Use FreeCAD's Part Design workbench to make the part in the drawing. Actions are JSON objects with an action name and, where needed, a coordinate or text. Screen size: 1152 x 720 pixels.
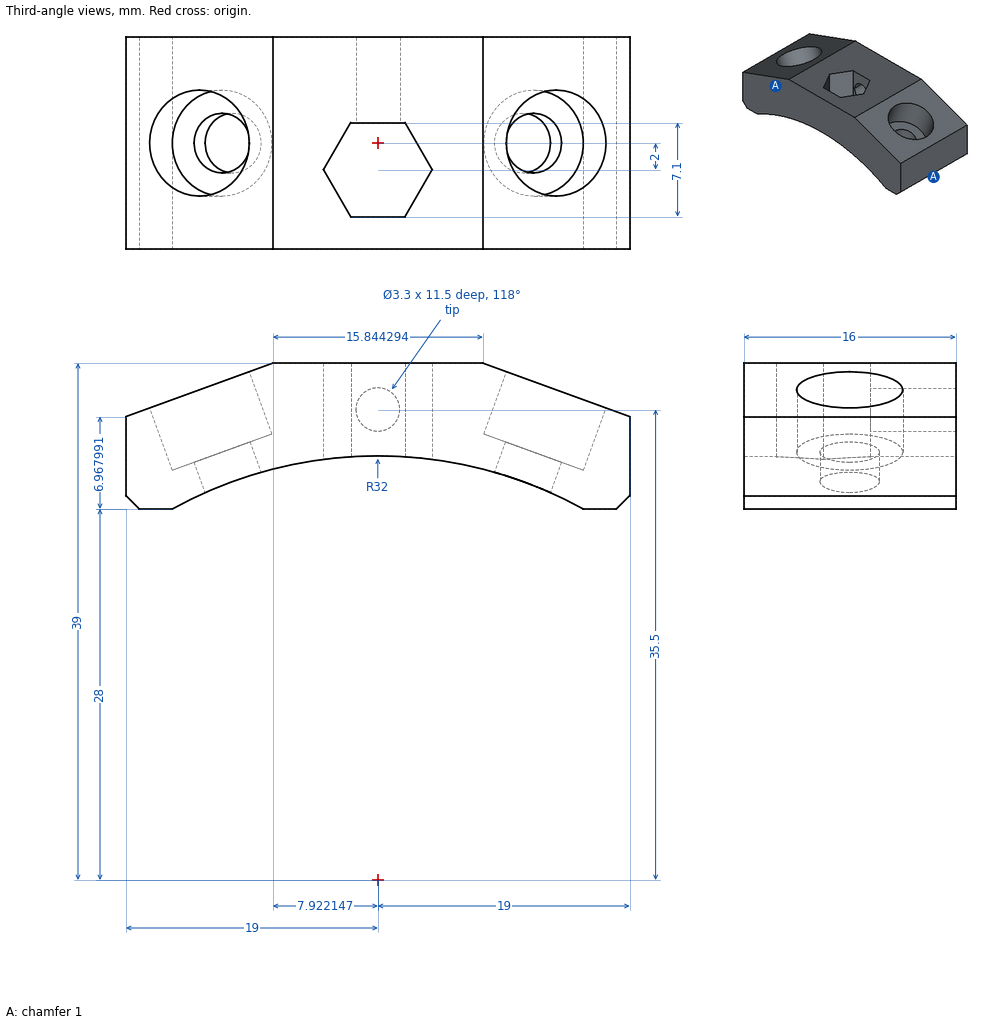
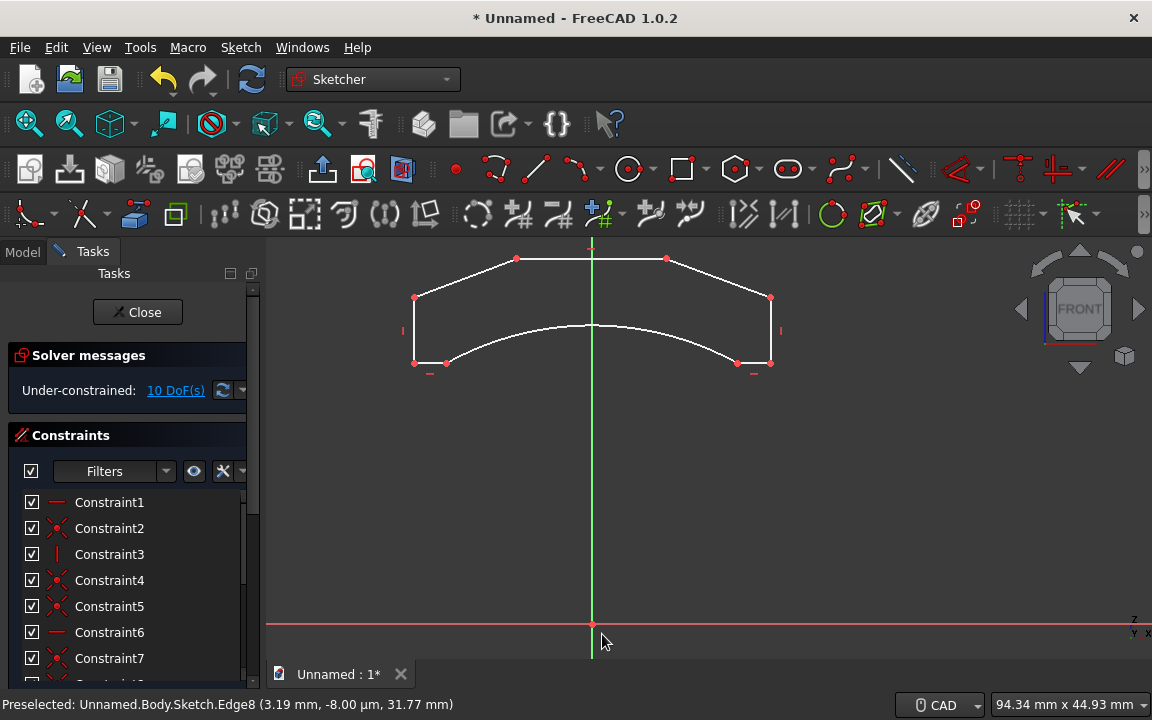
{"action": "key", "text": "d"}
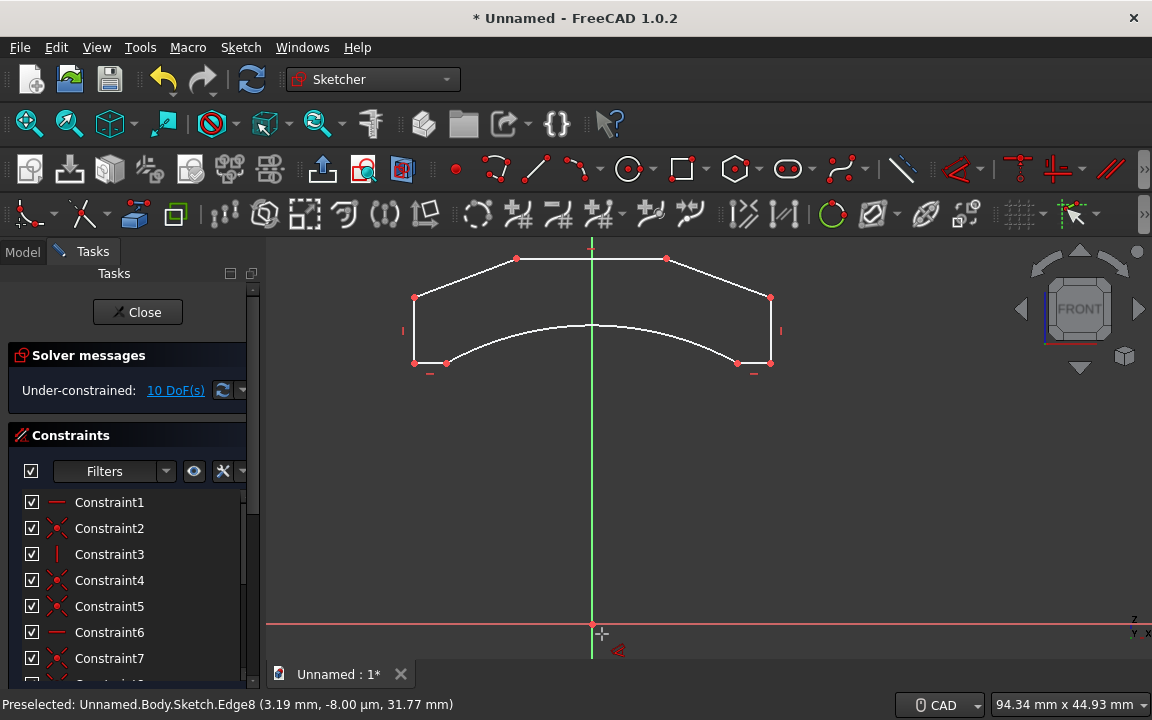
{"action": "left_click", "coordinate": [653, 332]}
{"action": "left_click", "coordinate": [660, 301]}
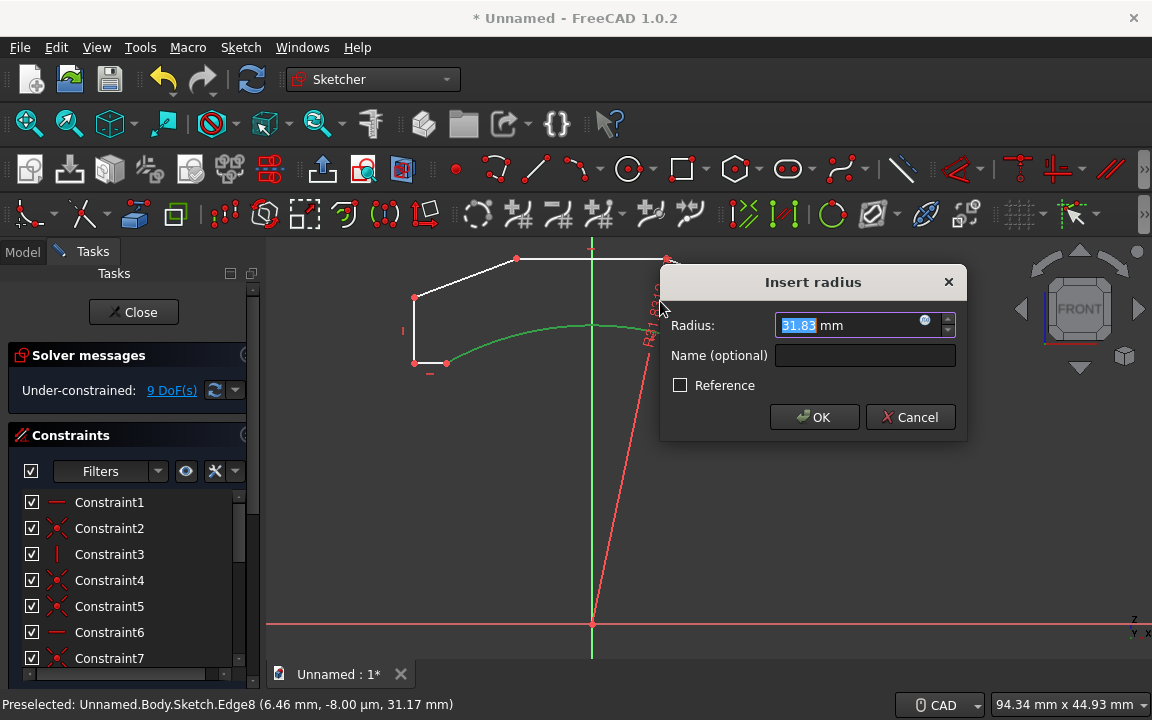
{"action": "type", "text": "32"}
{"action": "key", "text": "Return"}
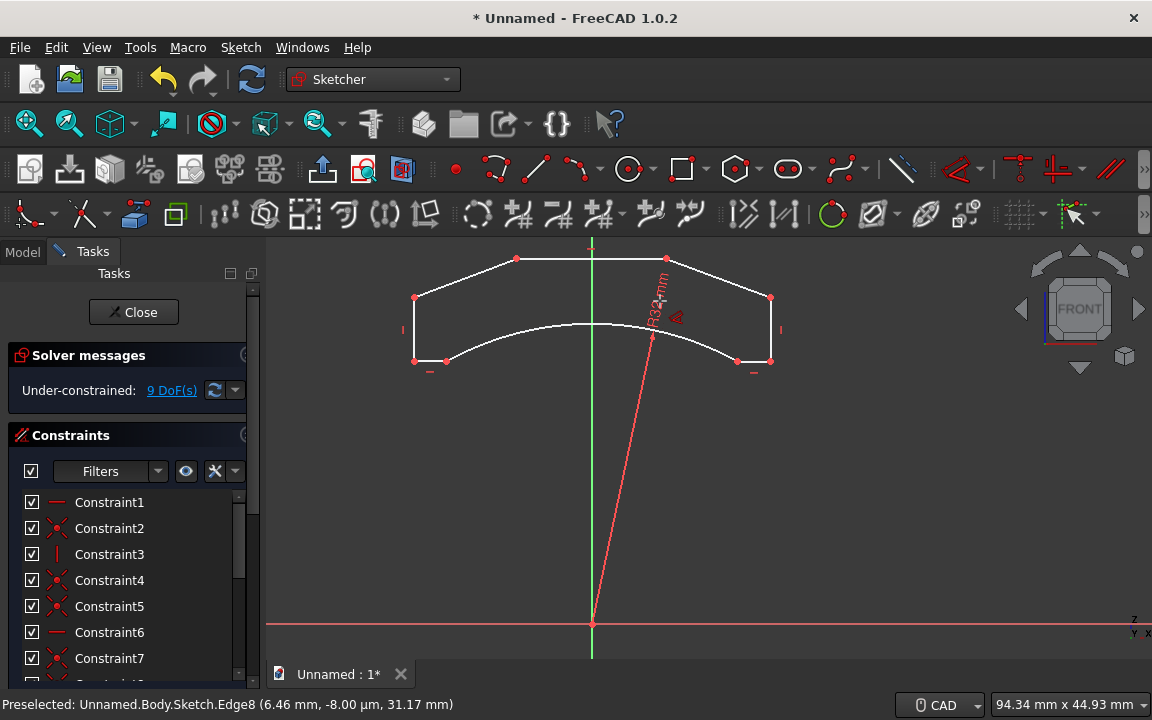
{"action": "left_click", "coordinate": [447, 361]}
{"action": "left_click", "coordinate": [413, 493]}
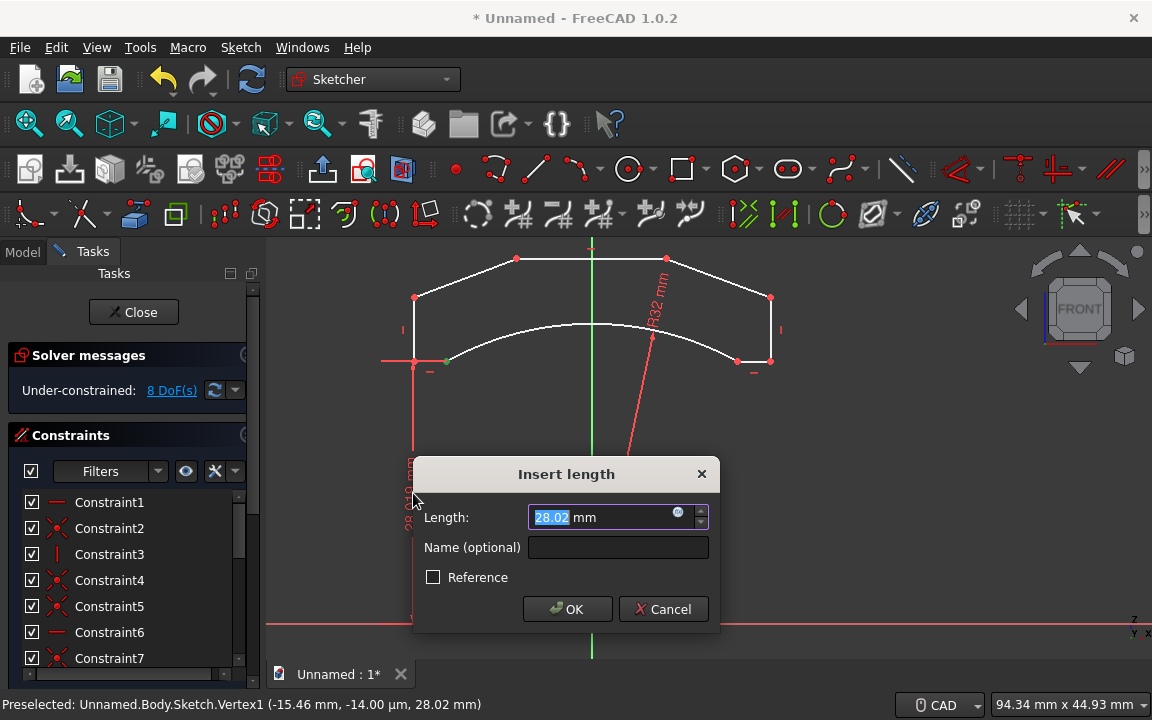
{"action": "type", "text": "28"}
{"action": "key", "text": "Return"}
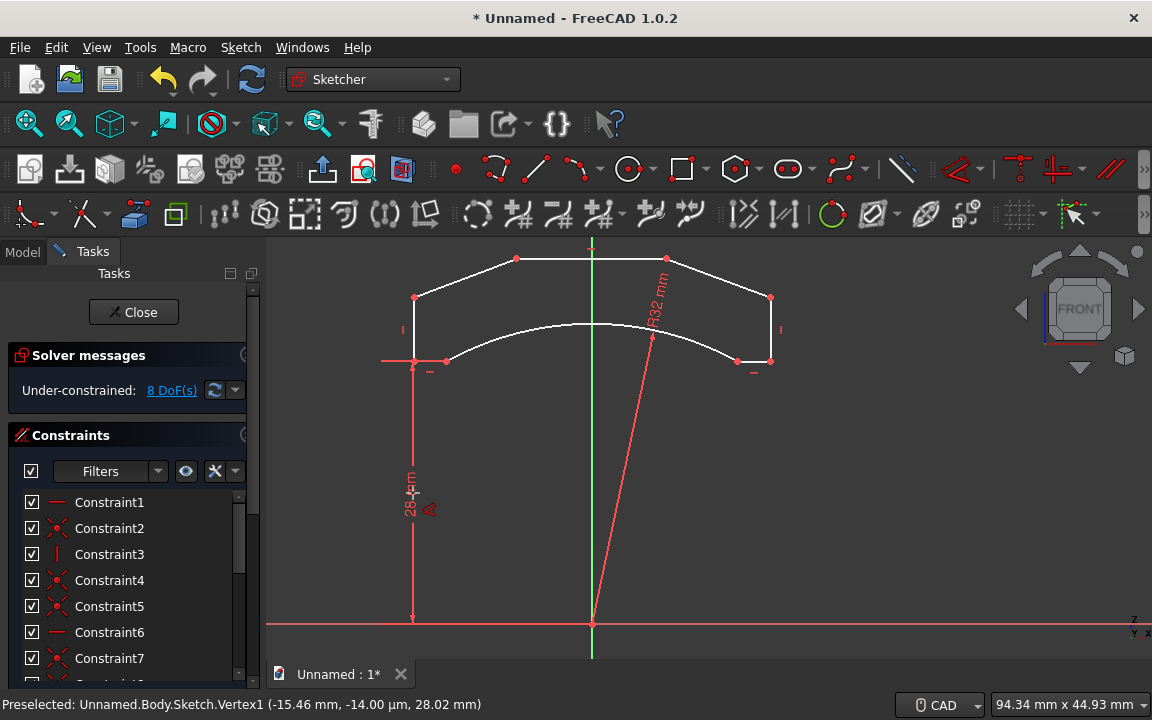
{"action": "left_click", "coordinate": [414, 361]}
{"action": "left_click", "coordinate": [462, 327]}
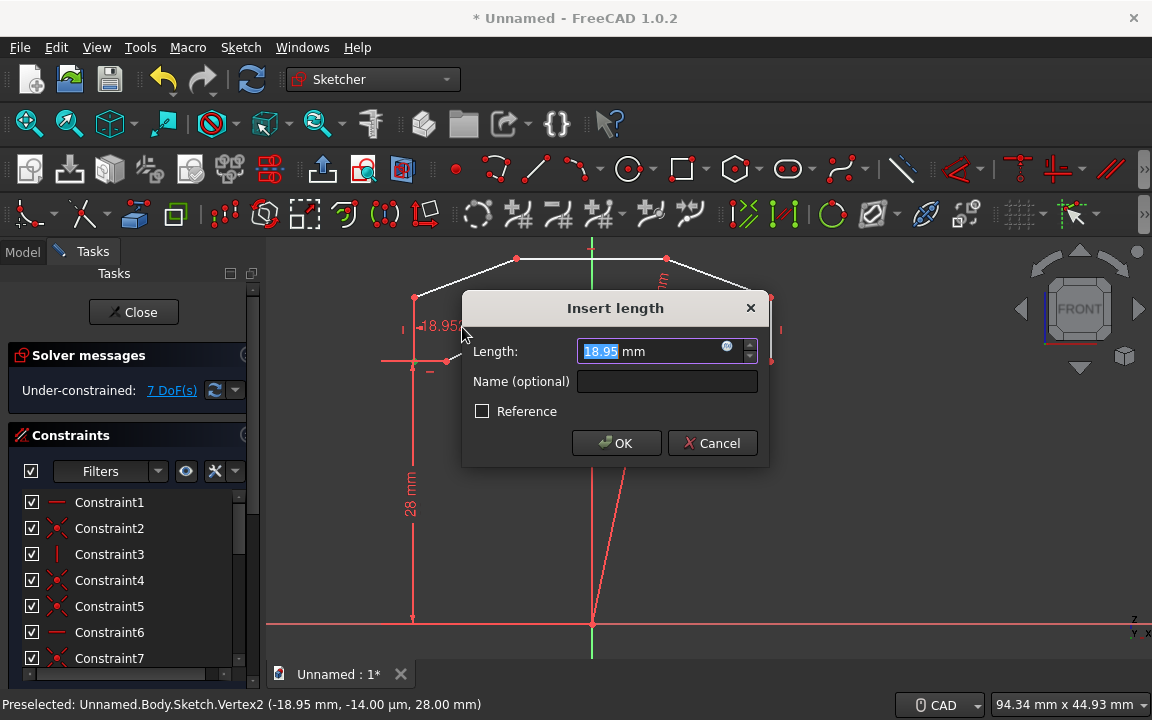
{"action": "type", "text": "19"}
{"action": "key", "text": "Return"}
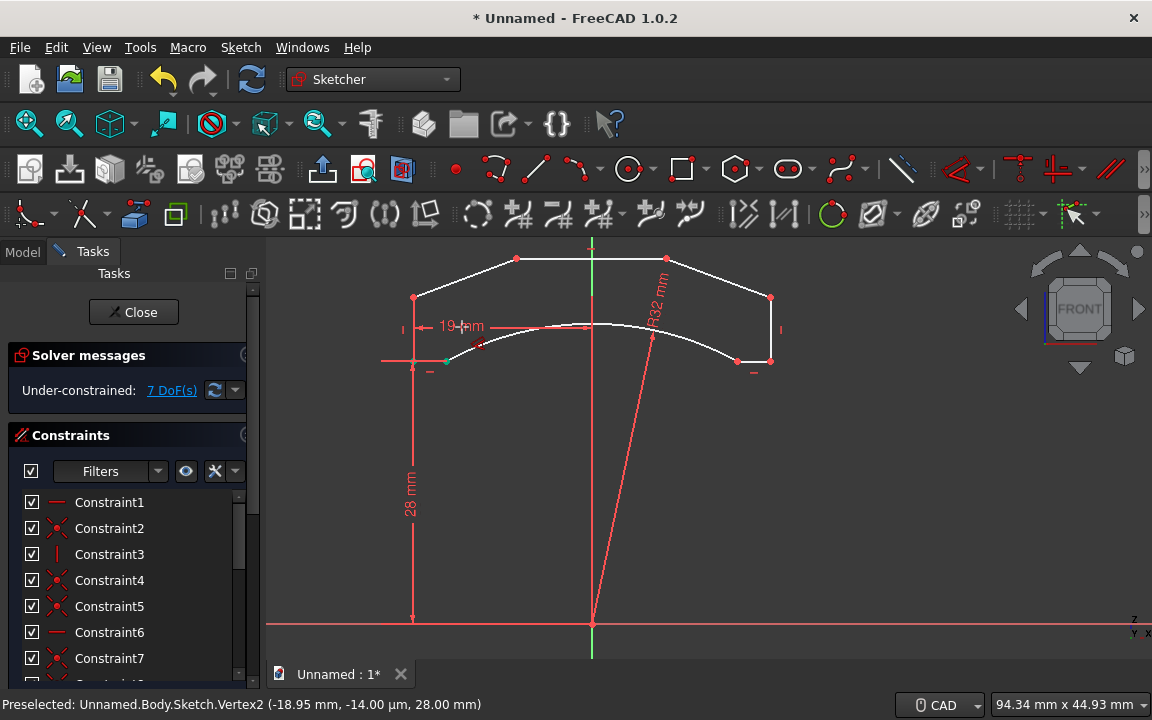
{"action": "scroll", "coordinate": [739, 462], "scroll_direction": "down", "scroll_amount": 2}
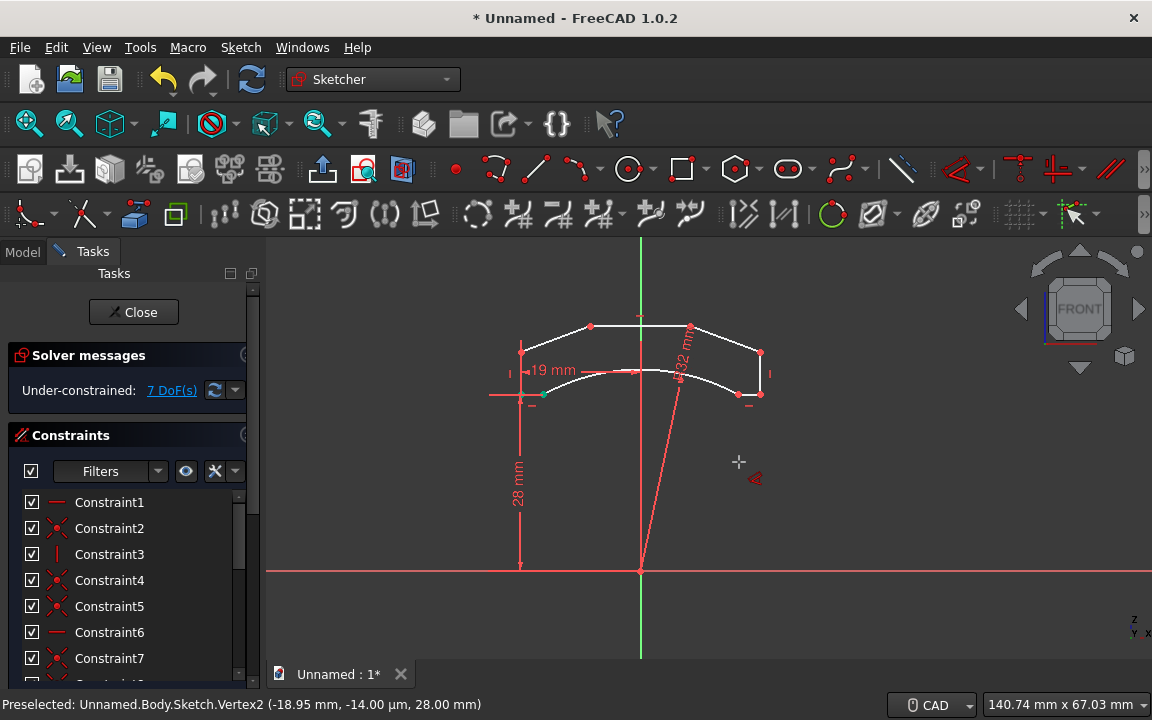
{"action": "left_click", "coordinate": [590, 326]}
{"action": "left_click", "coordinate": [556, 449]}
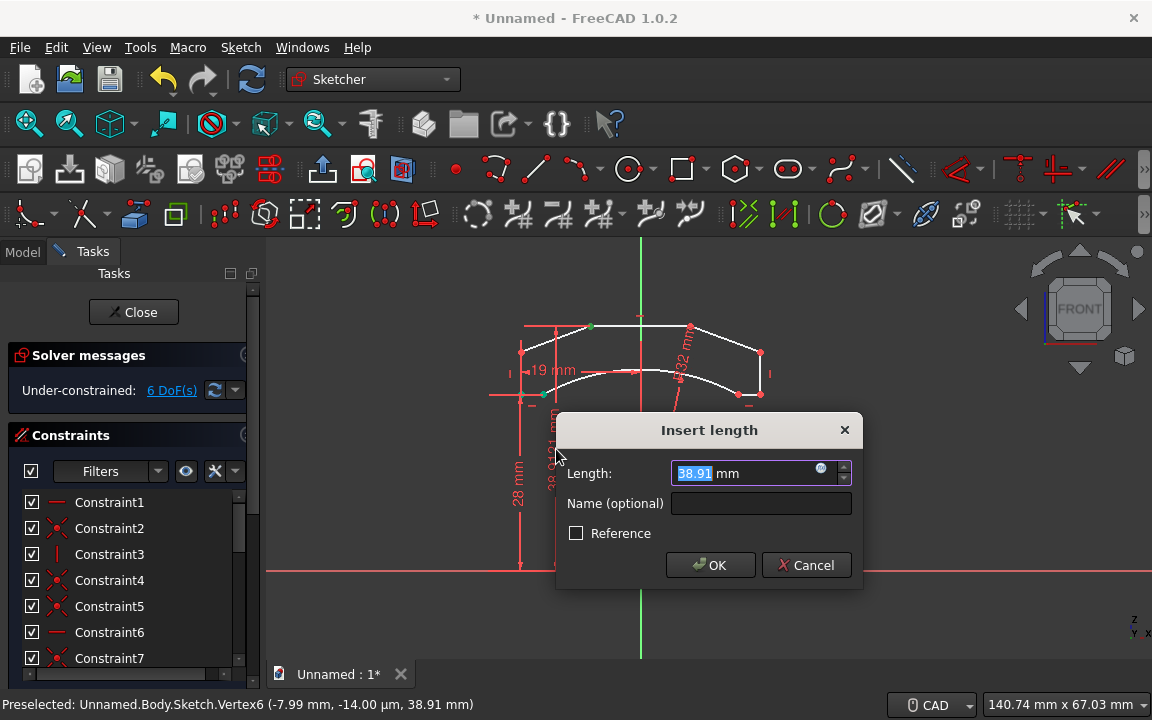
{"action": "type", "text": "39"}
{"action": "key", "text": "Return"}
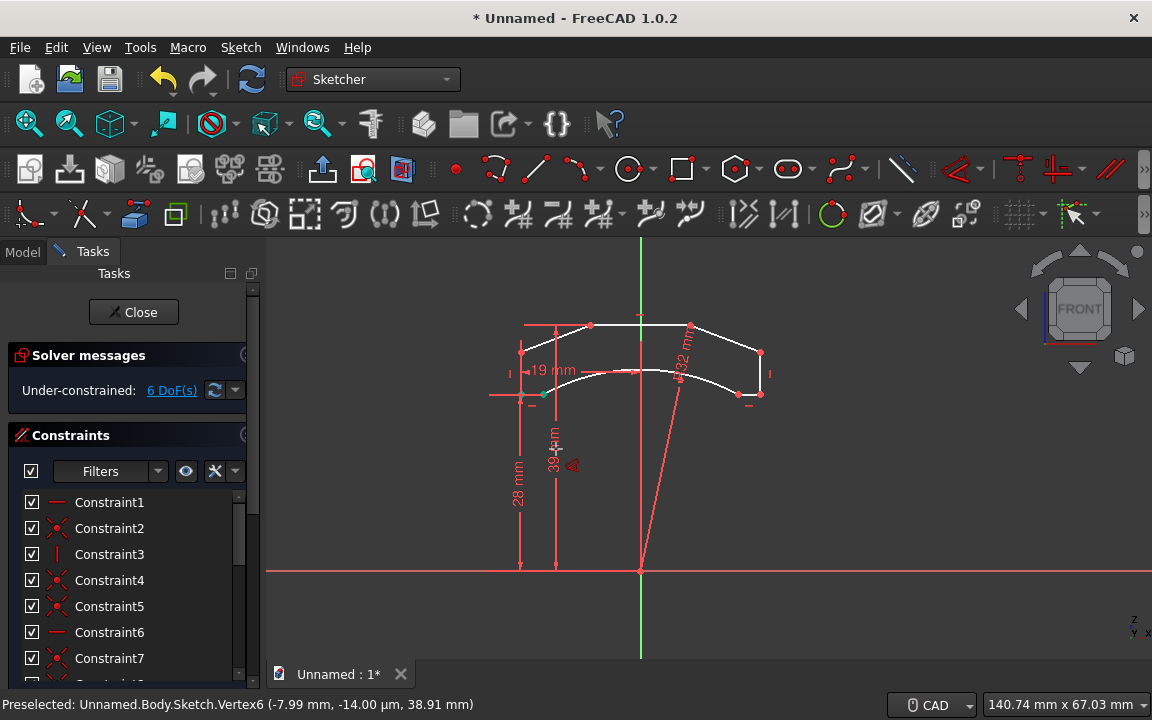
{"action": "left_click", "coordinate": [760, 352]}
{"action": "left_click", "coordinate": [700, 605]}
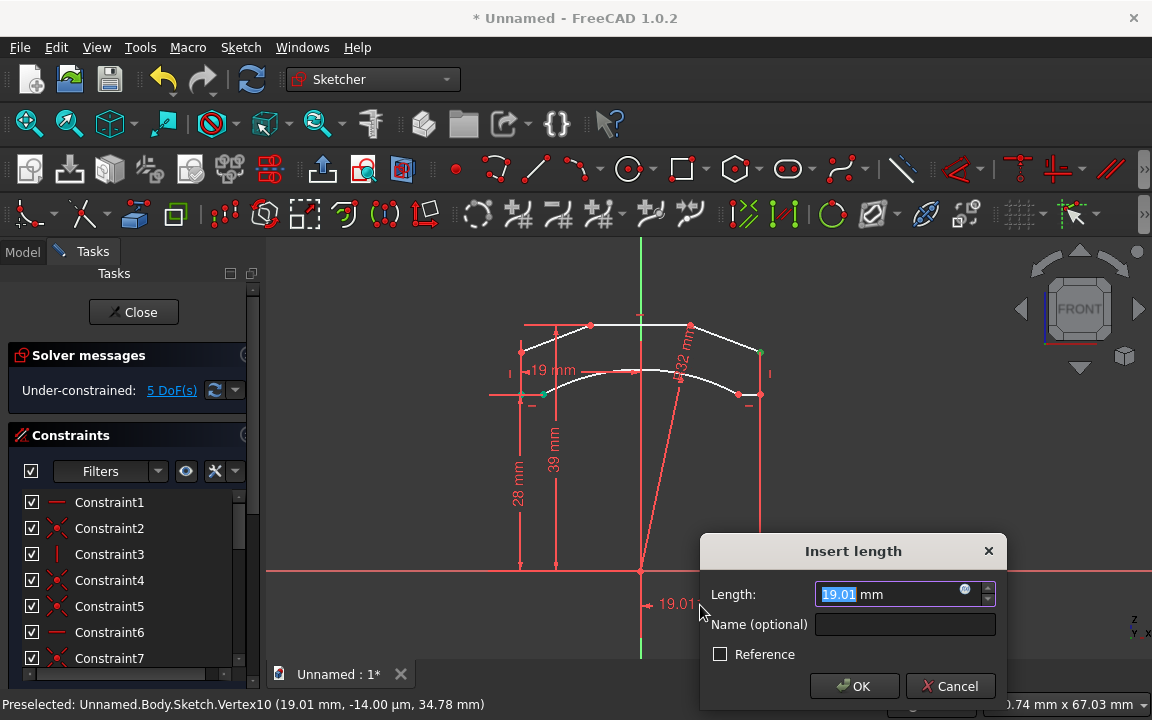
{"action": "type", "text": "19"}
{"action": "key", "text": "Return"}